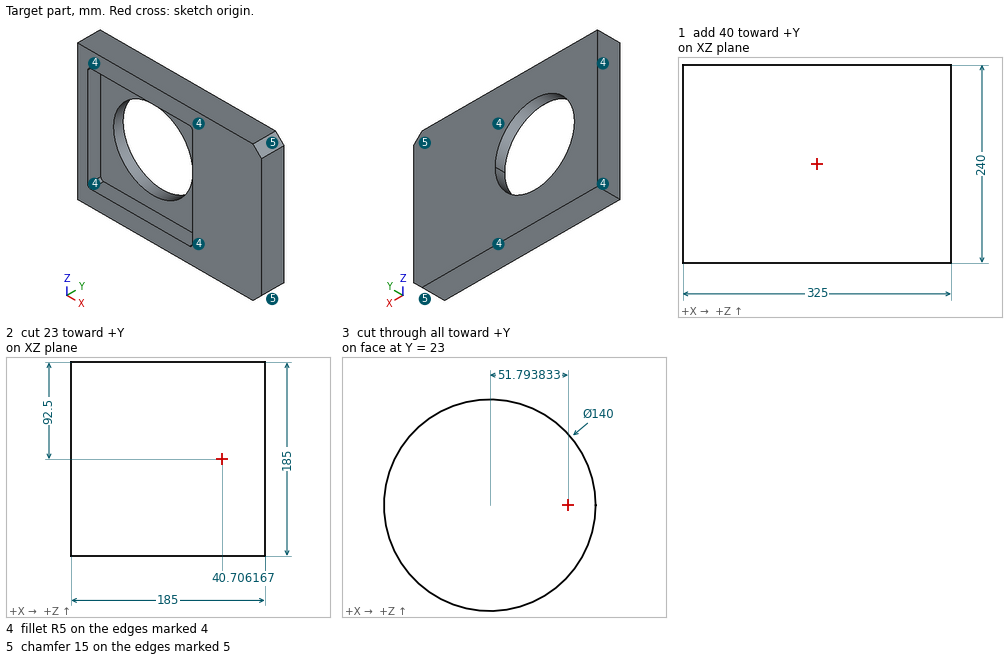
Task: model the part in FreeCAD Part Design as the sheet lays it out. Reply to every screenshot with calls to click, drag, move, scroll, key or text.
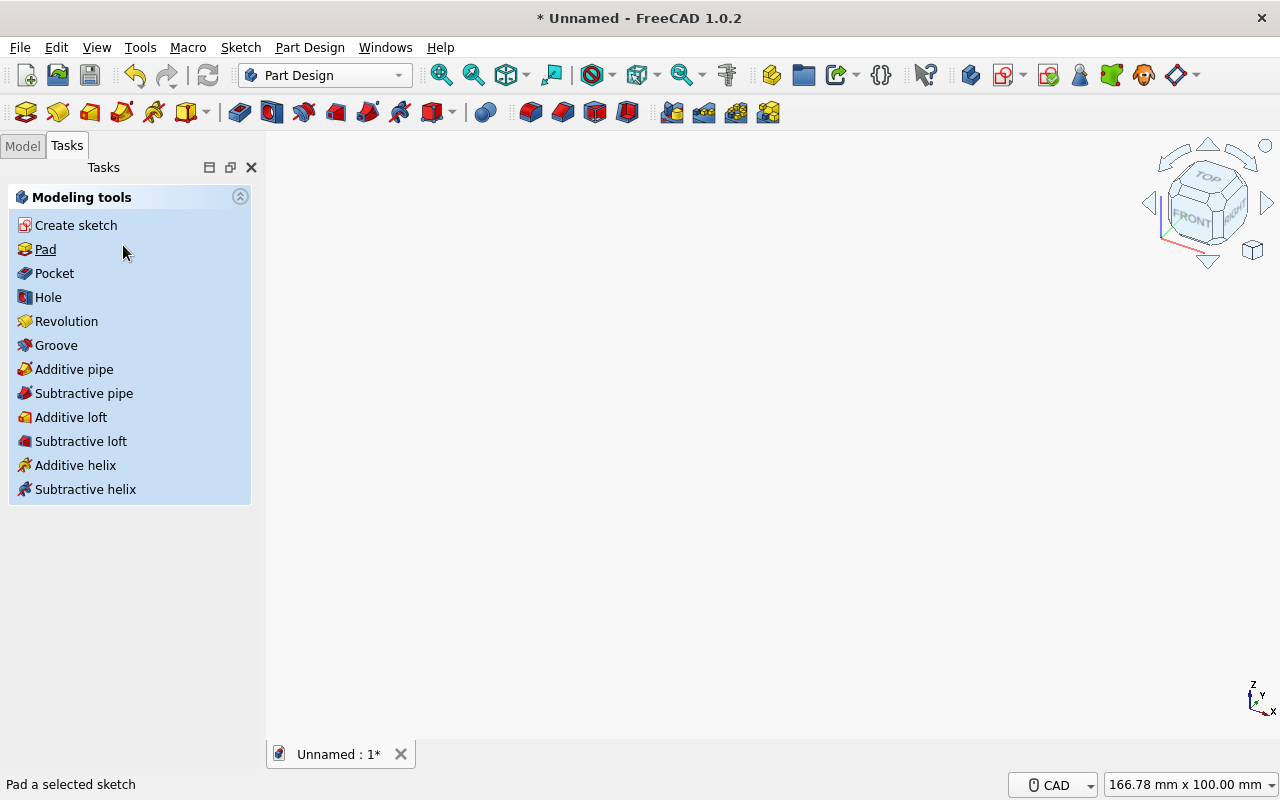
click(26, 112)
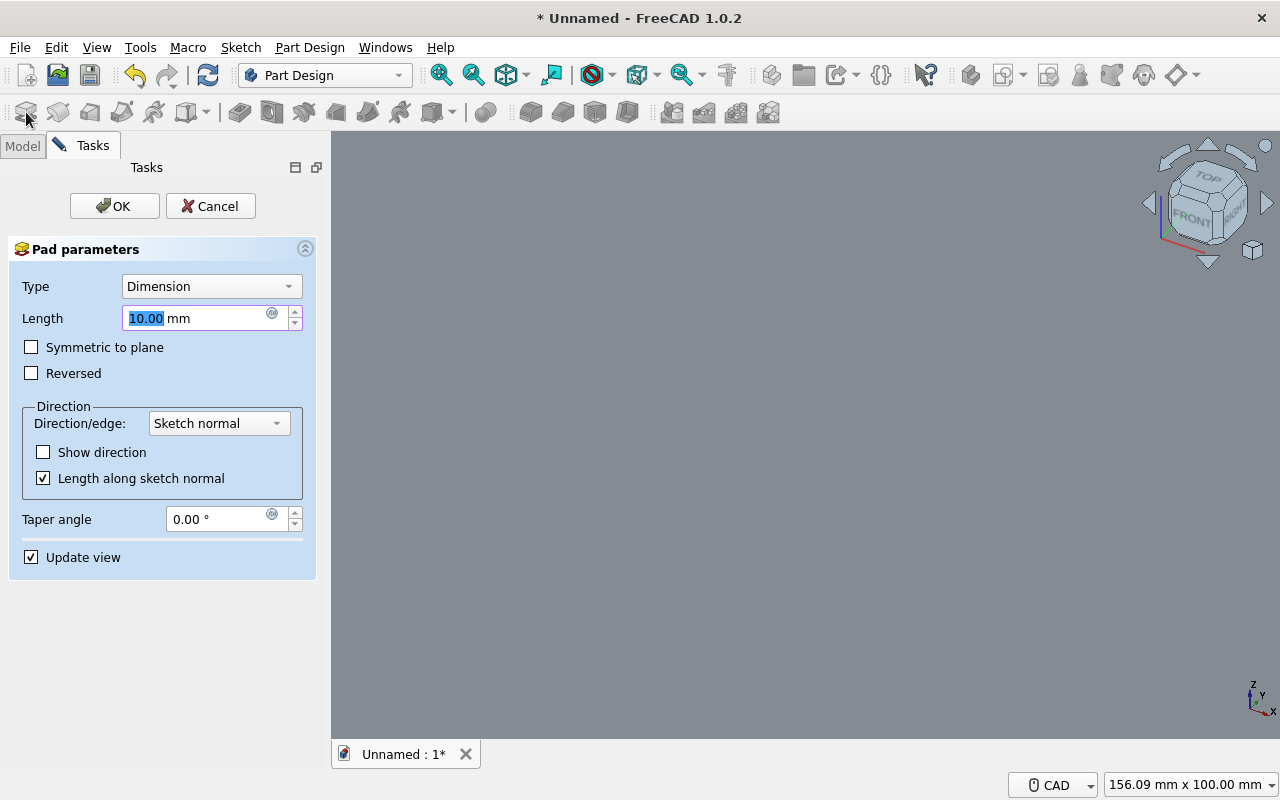
text(40)
key(Tab)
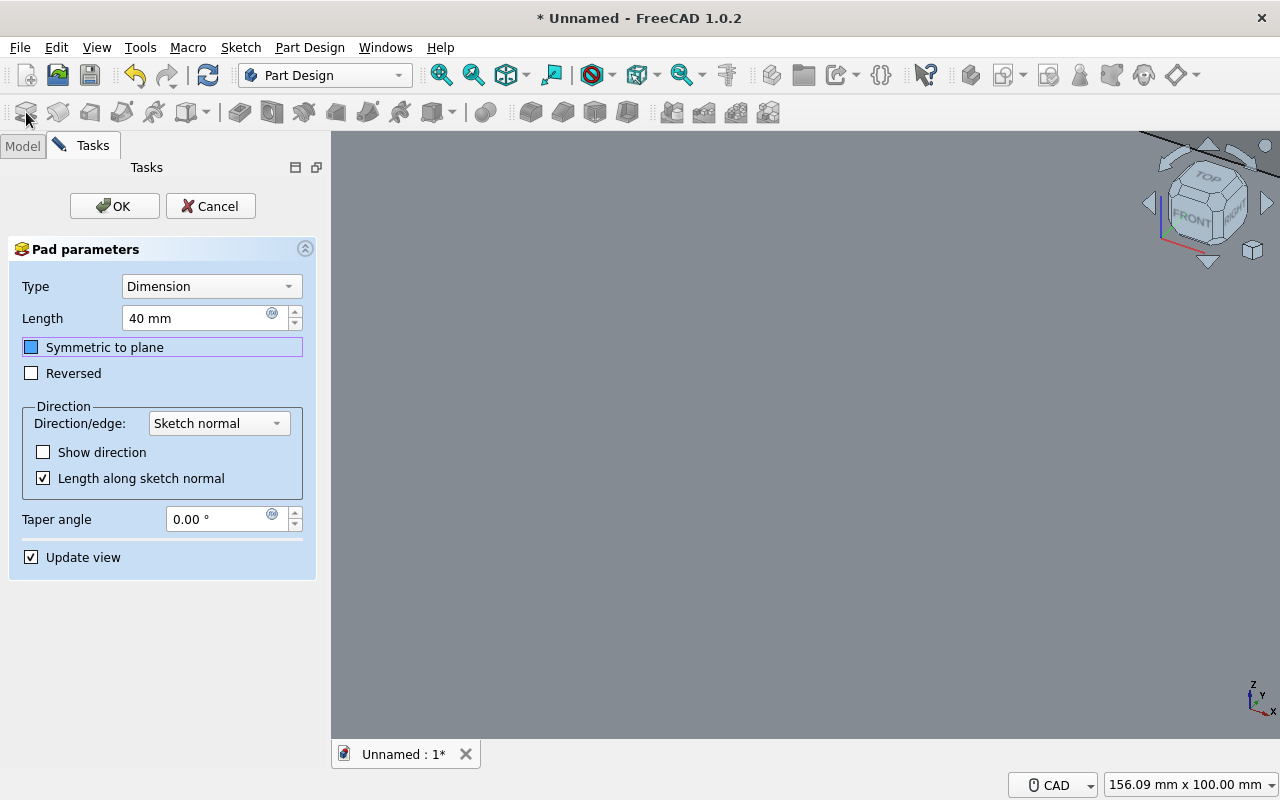
click(30, 373)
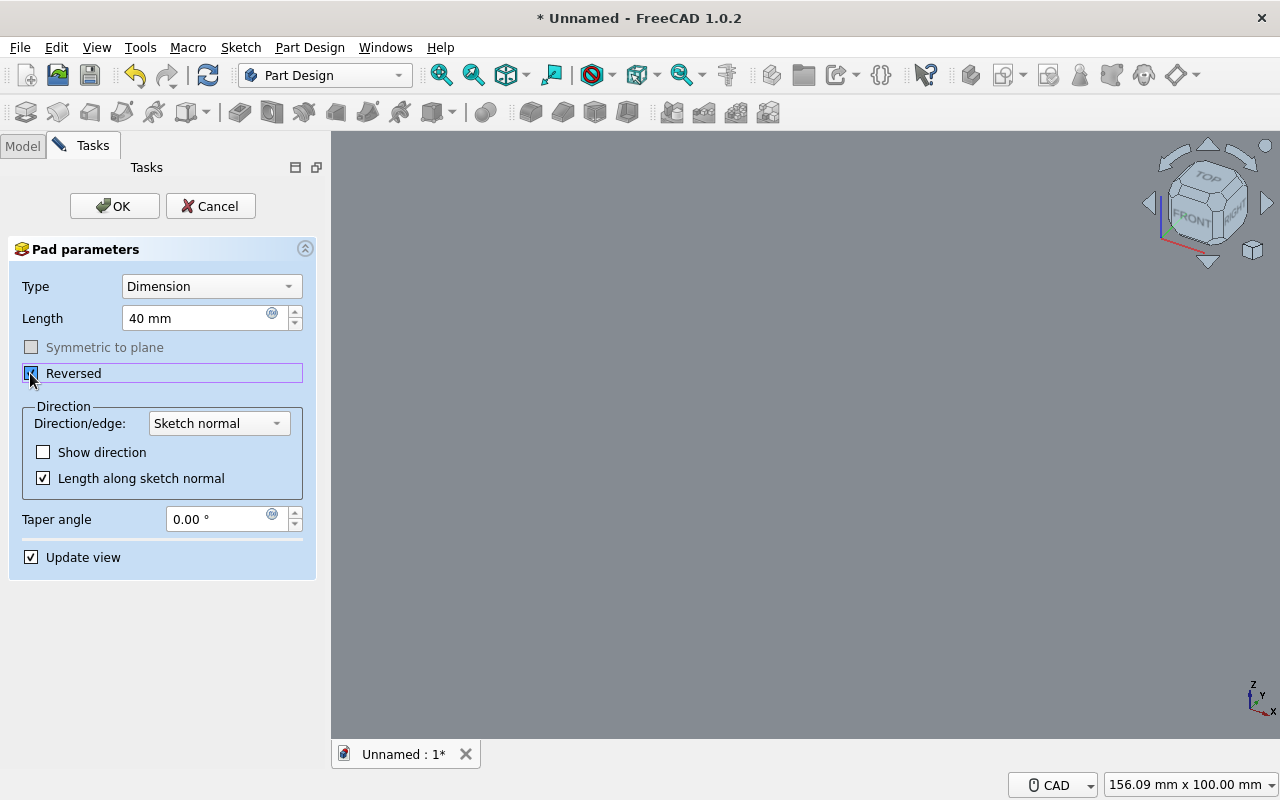
click(115, 206)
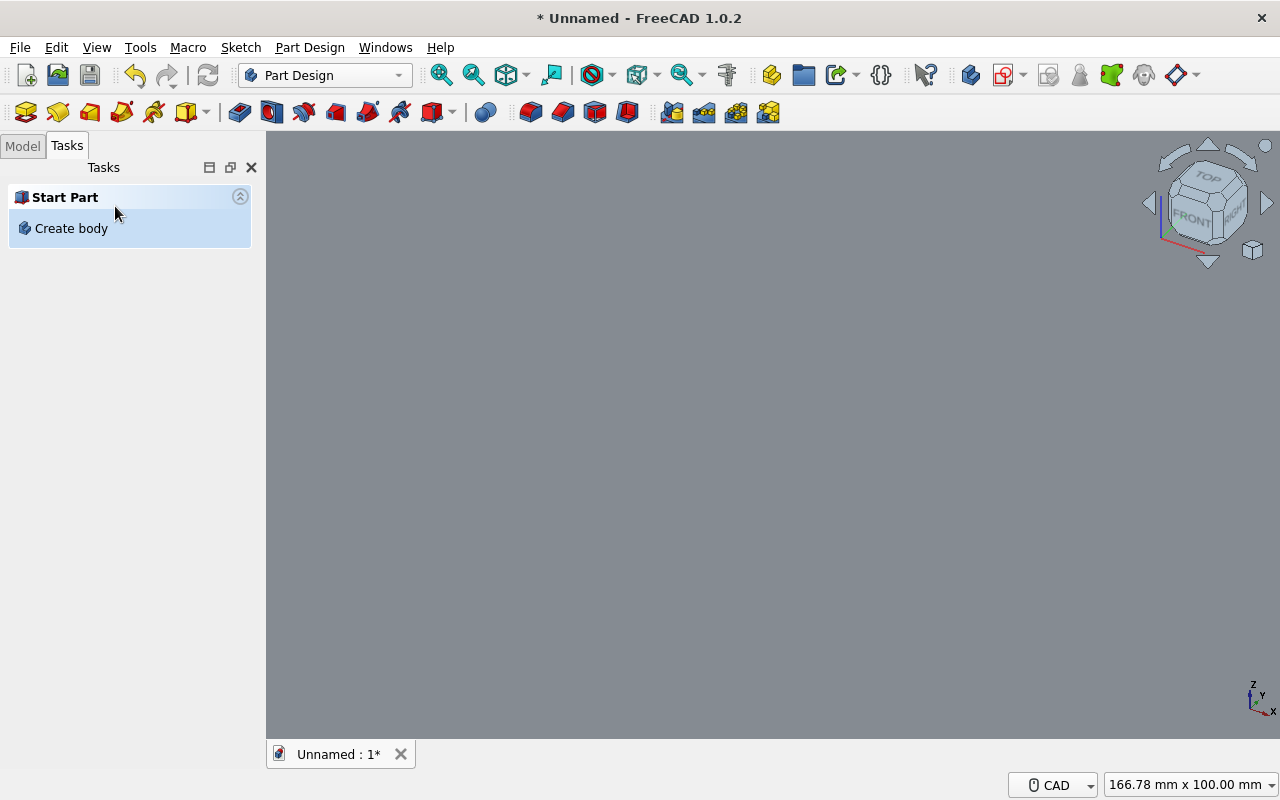
click(442, 76)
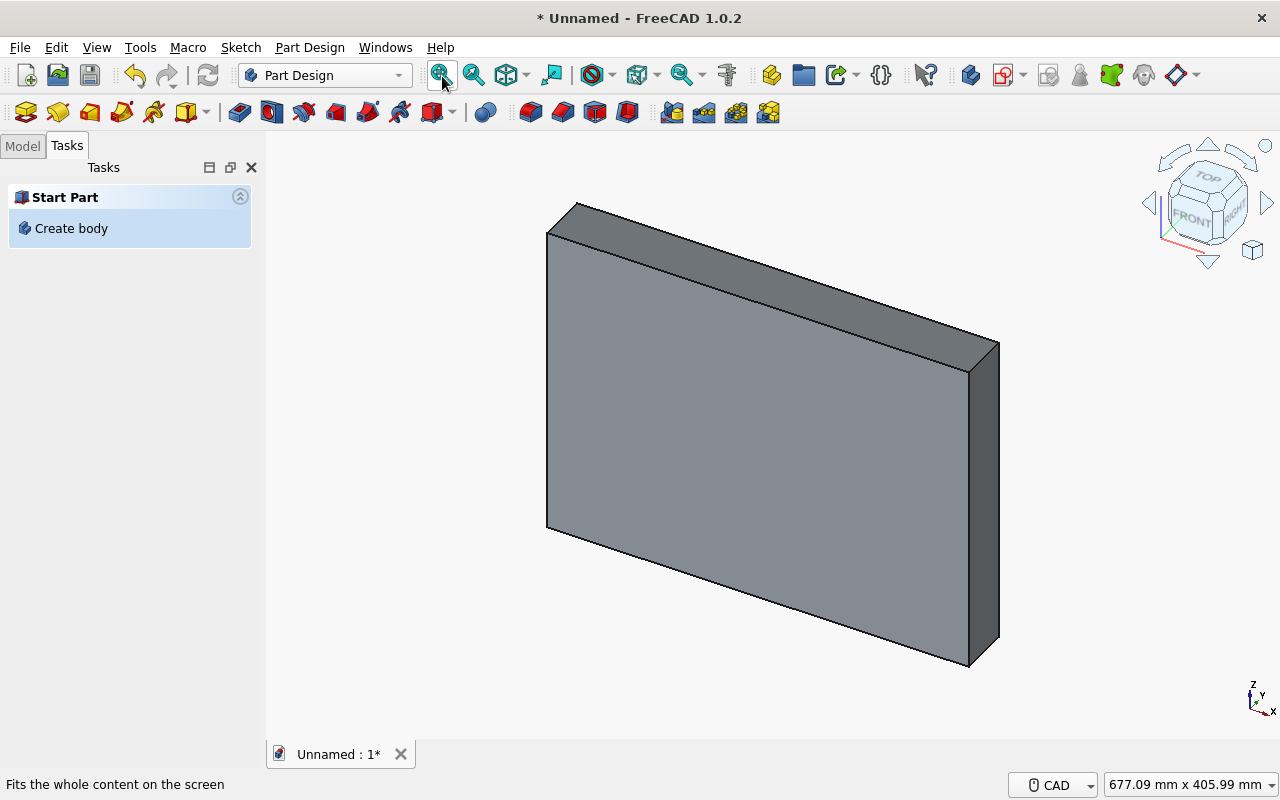
click(1004, 76)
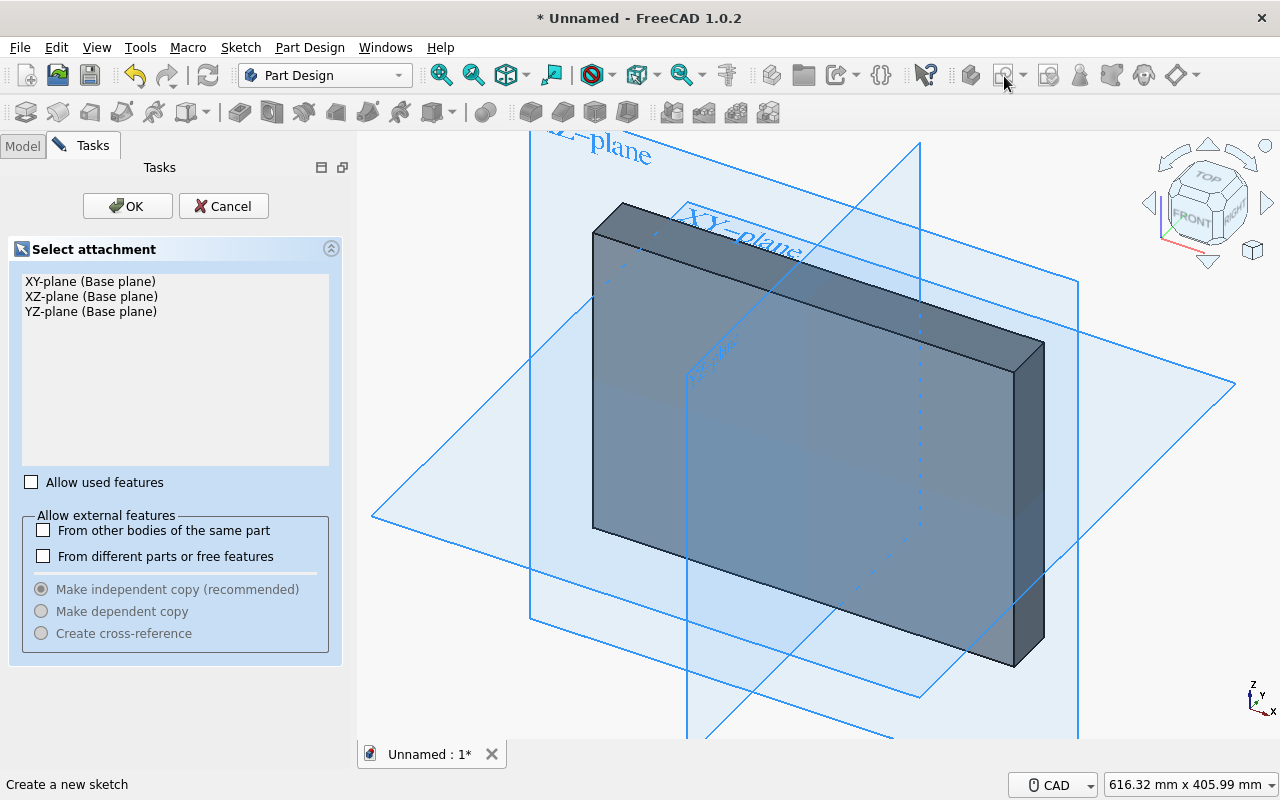
click(82, 296)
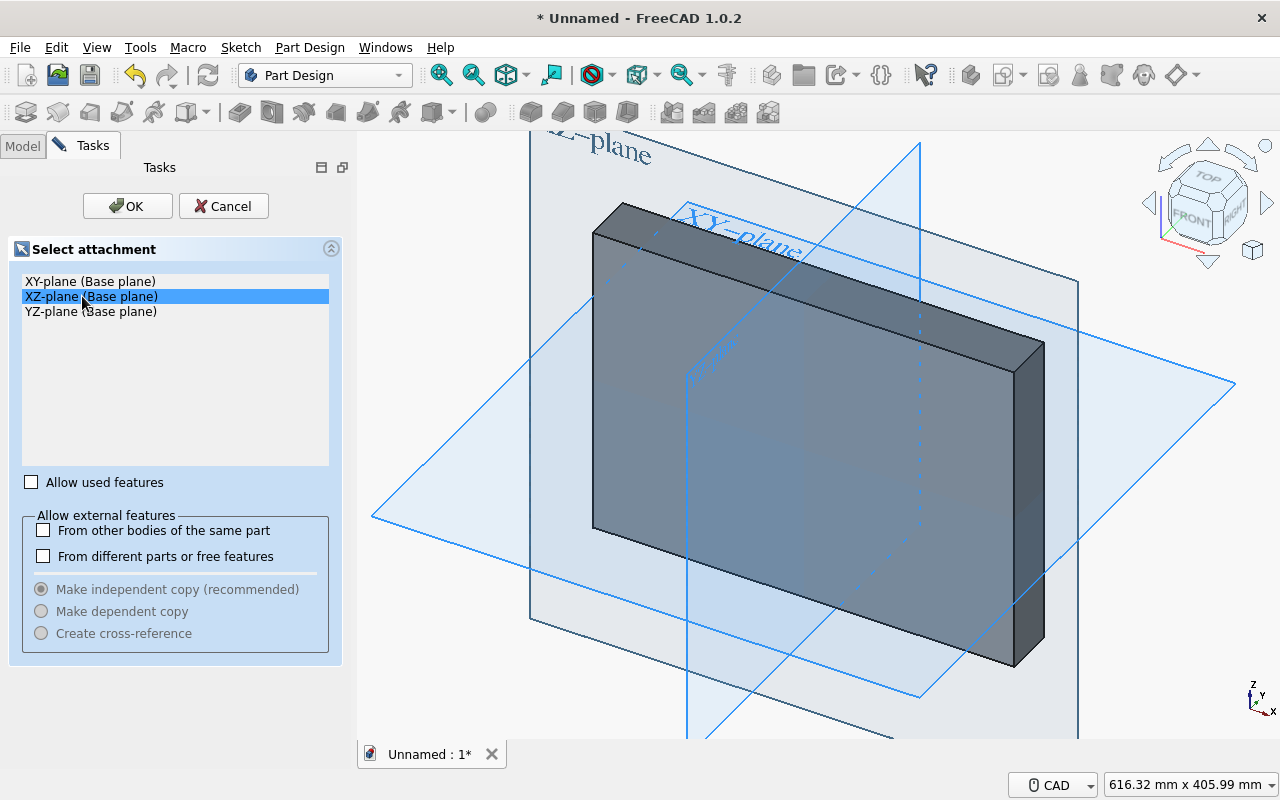
click(128, 206)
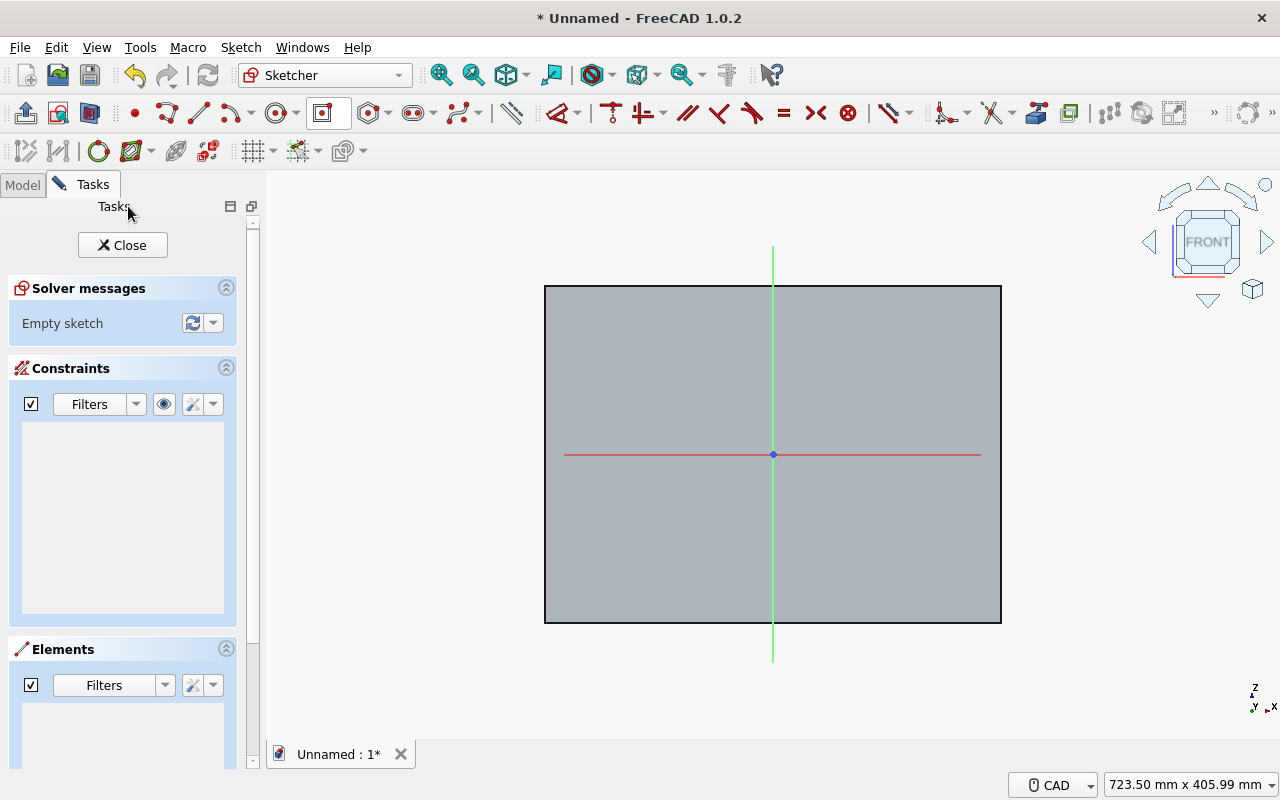
scroll(692, 455, up, 2)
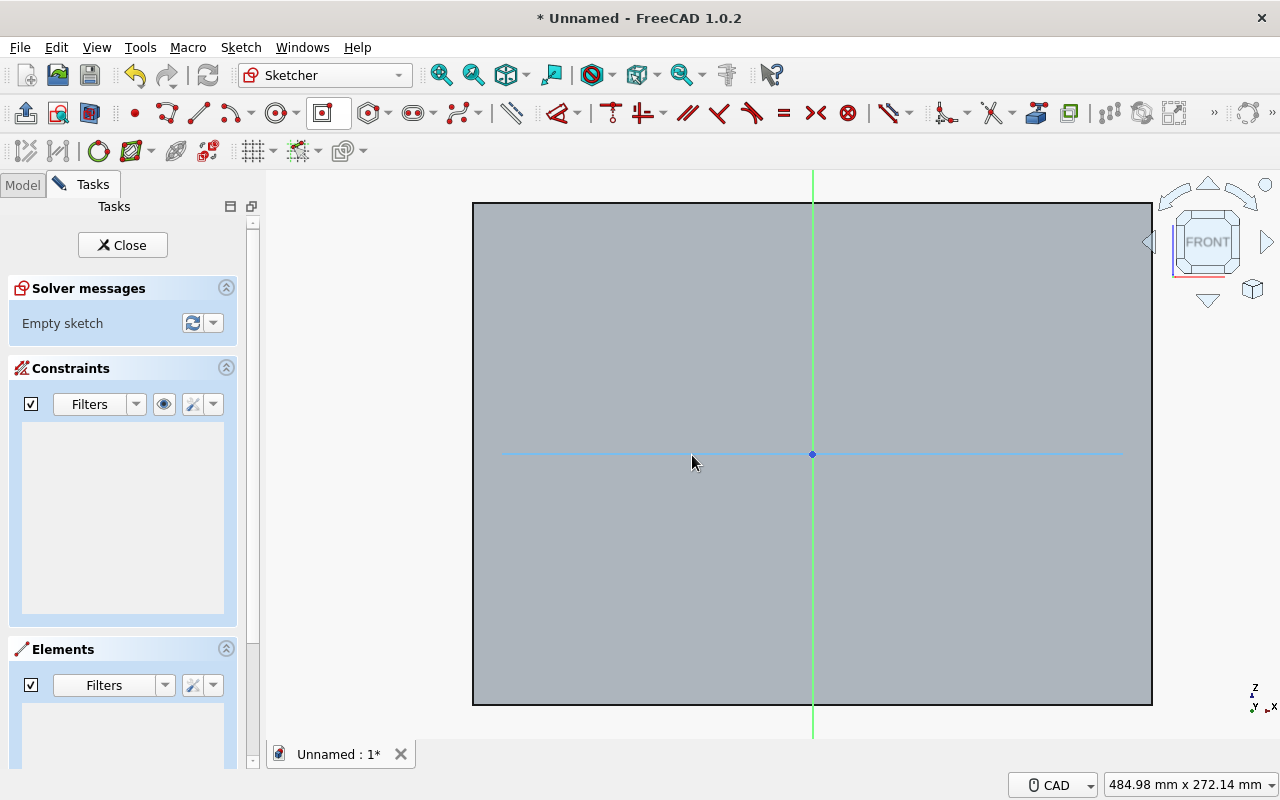
key(g)
key(r)